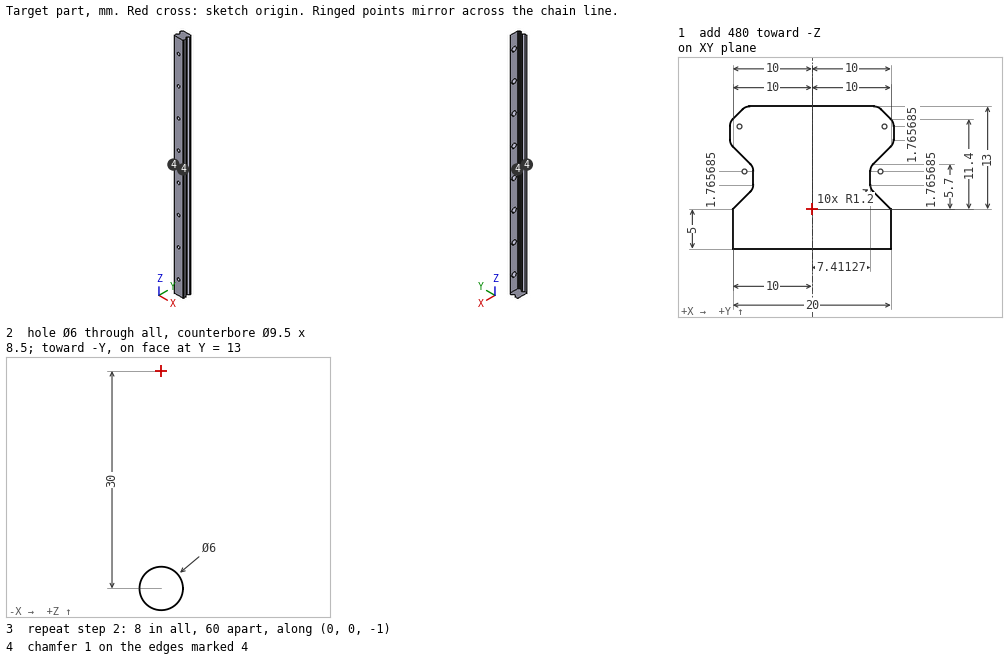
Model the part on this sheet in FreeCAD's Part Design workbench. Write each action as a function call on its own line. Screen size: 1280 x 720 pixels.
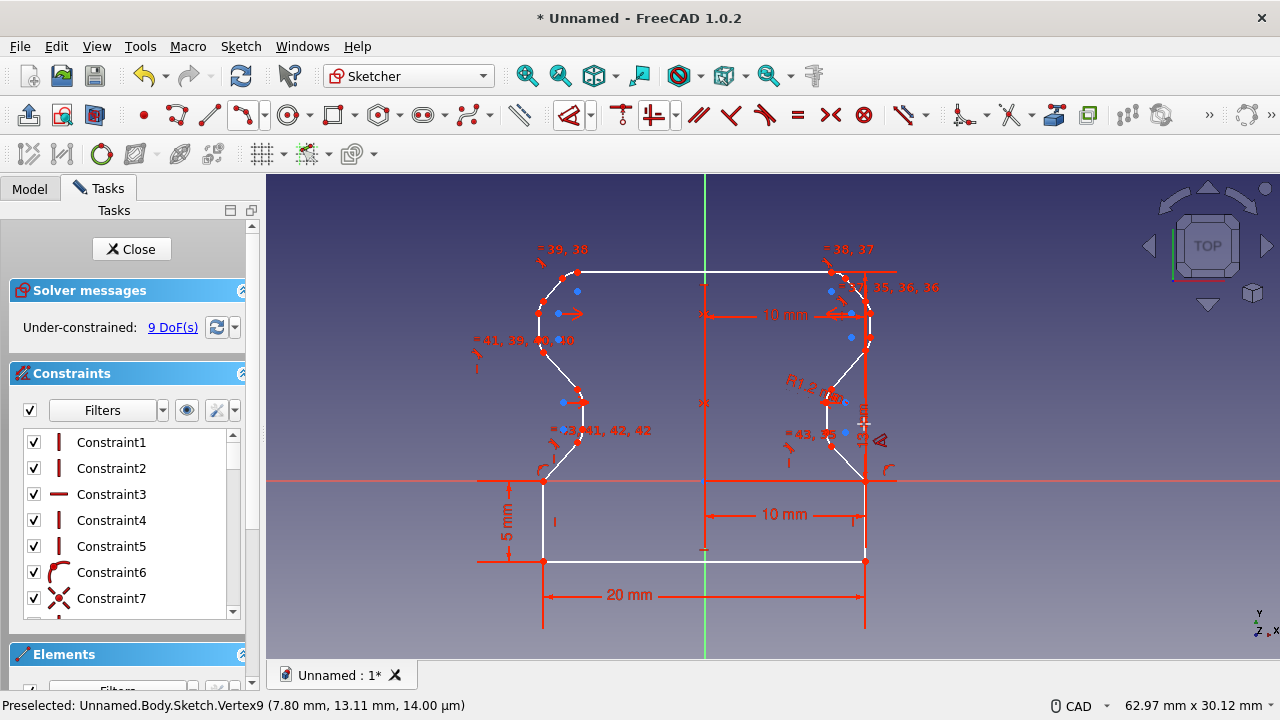
click(543, 301)
click(624, 515)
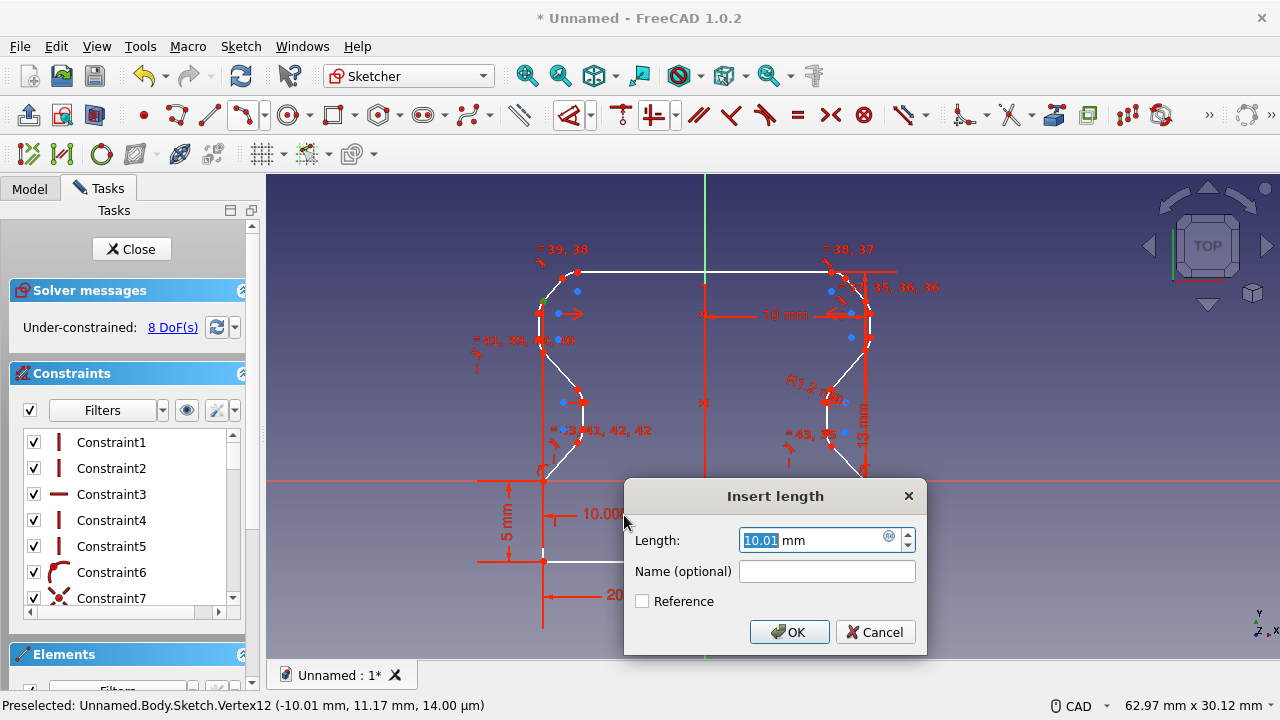
text(10)
key(Return)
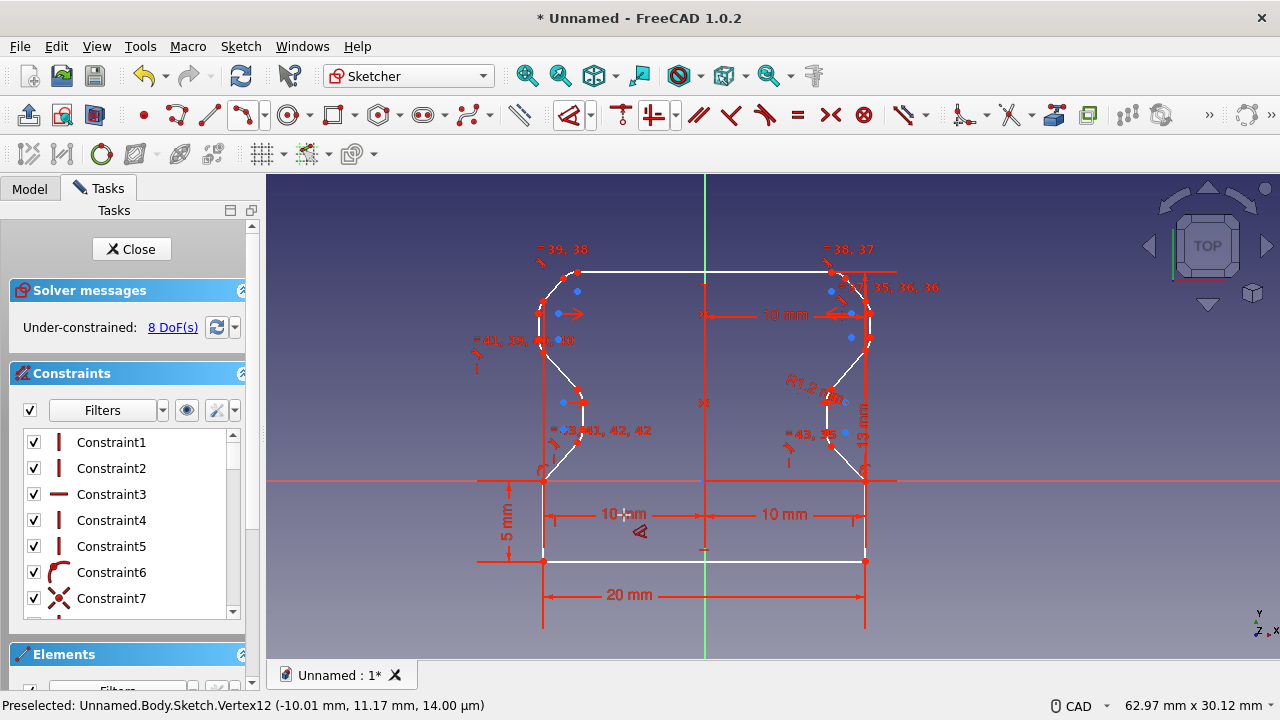
click(544, 352)
click(624, 318)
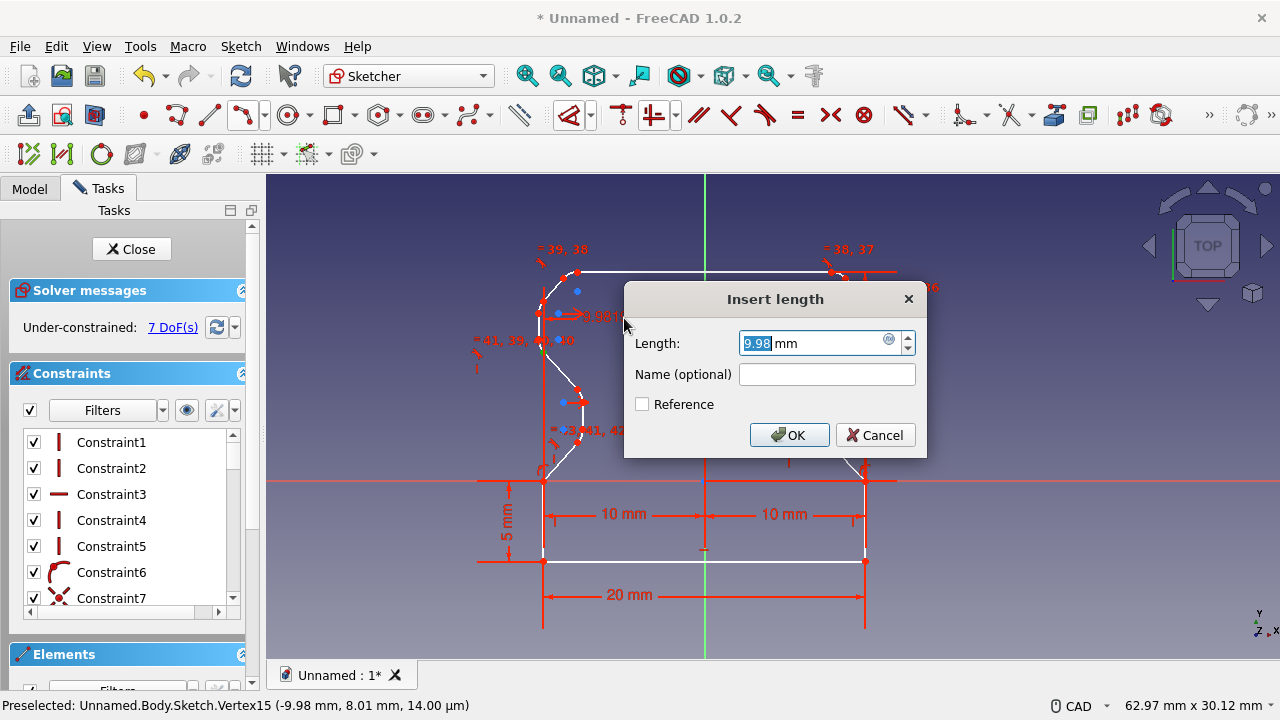
text(10)
key(Return)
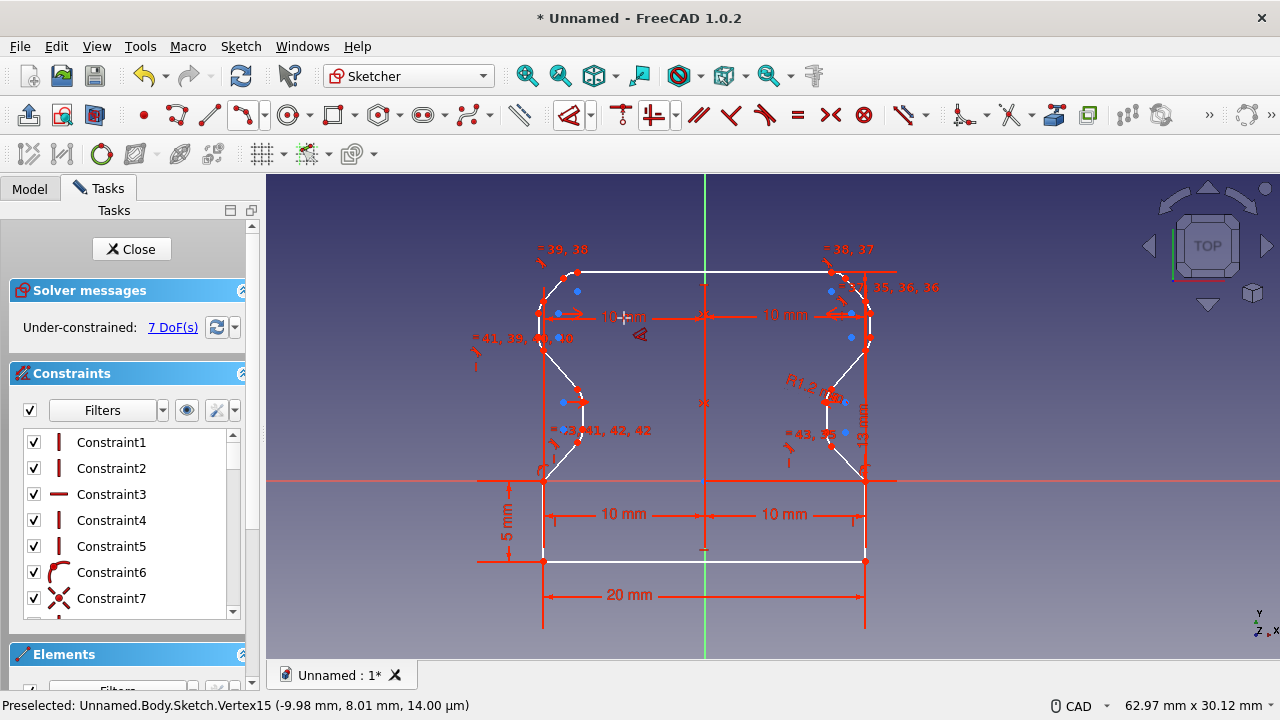
click(543, 481)
click(624, 447)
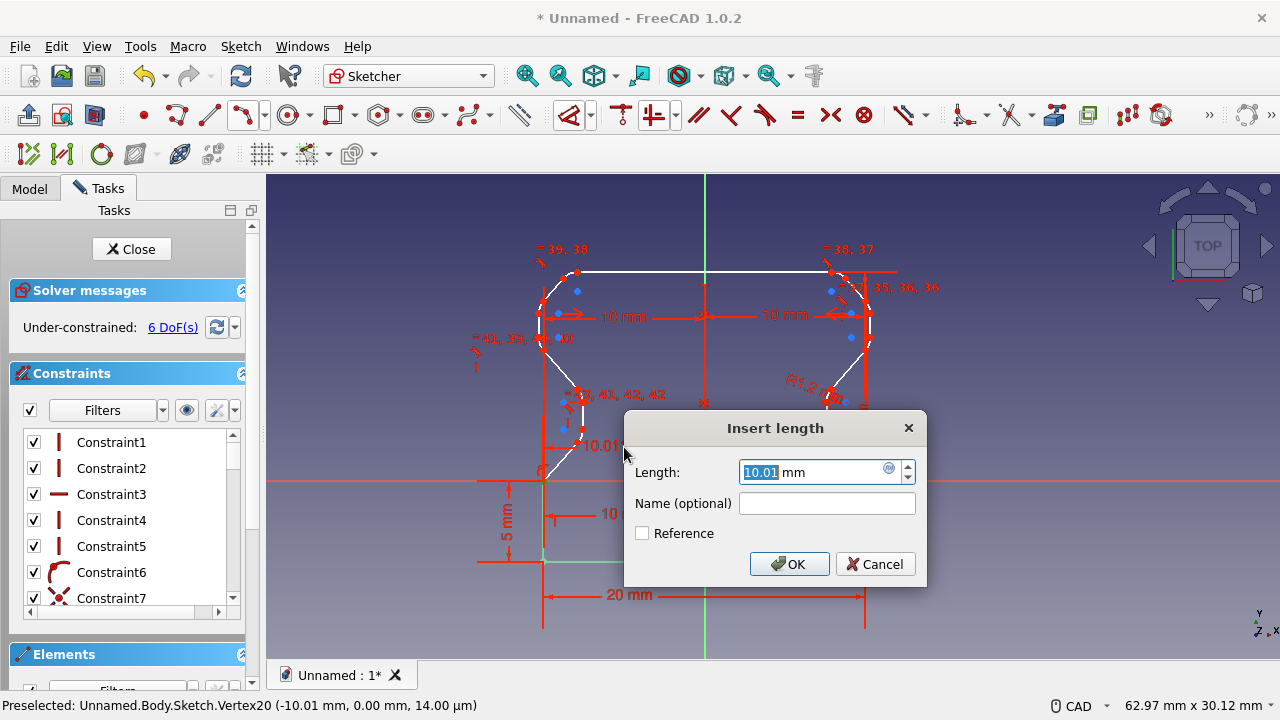
text(10)
key(Return)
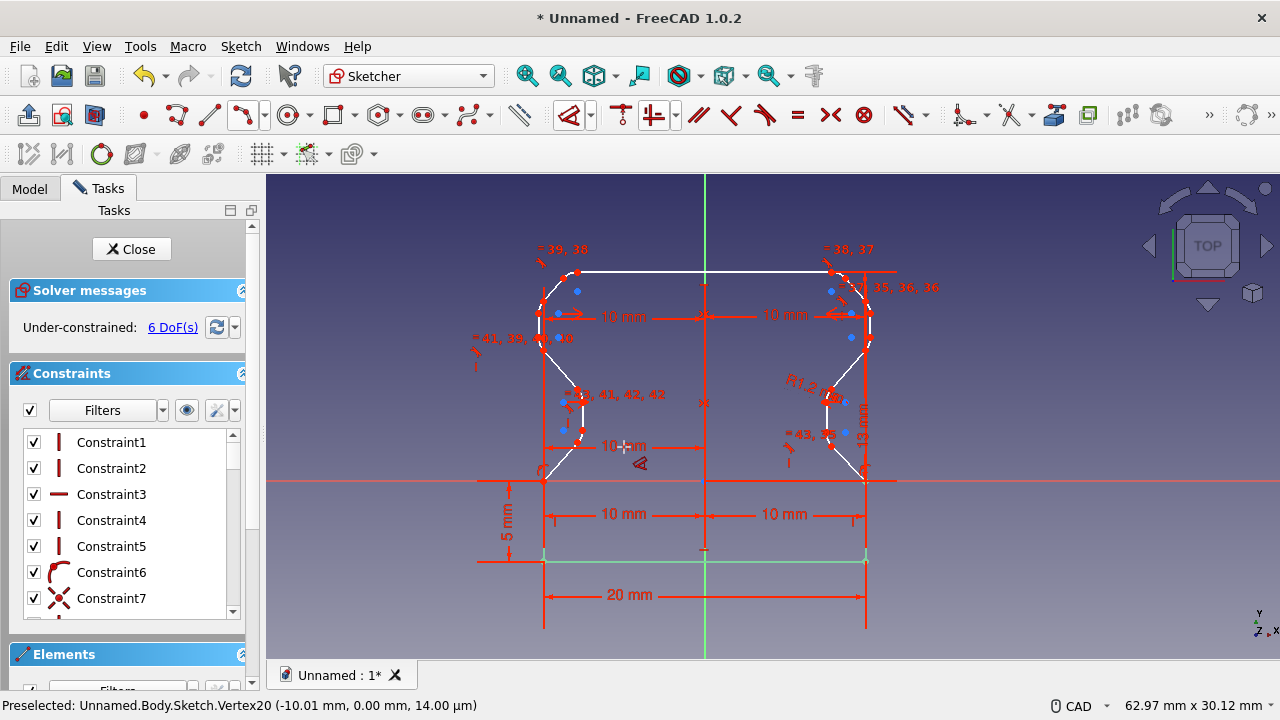
click(831, 390)
click(865, 457)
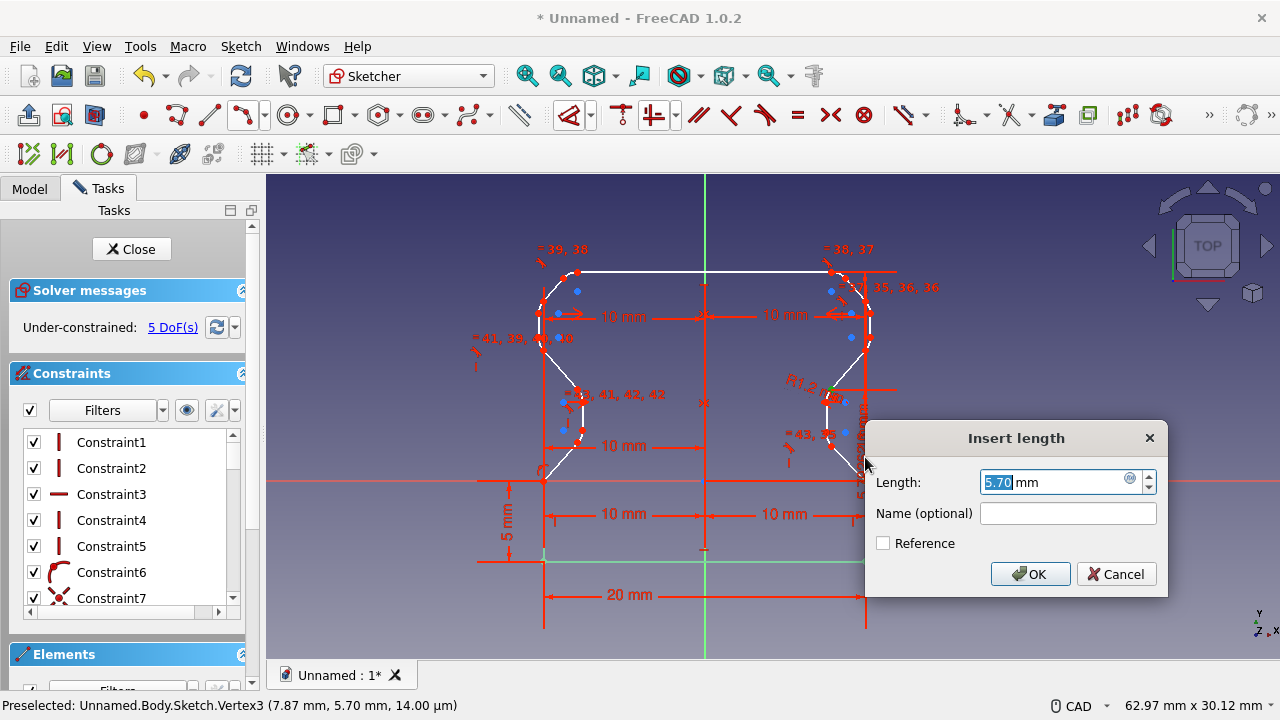
text(5.7)
key(Return)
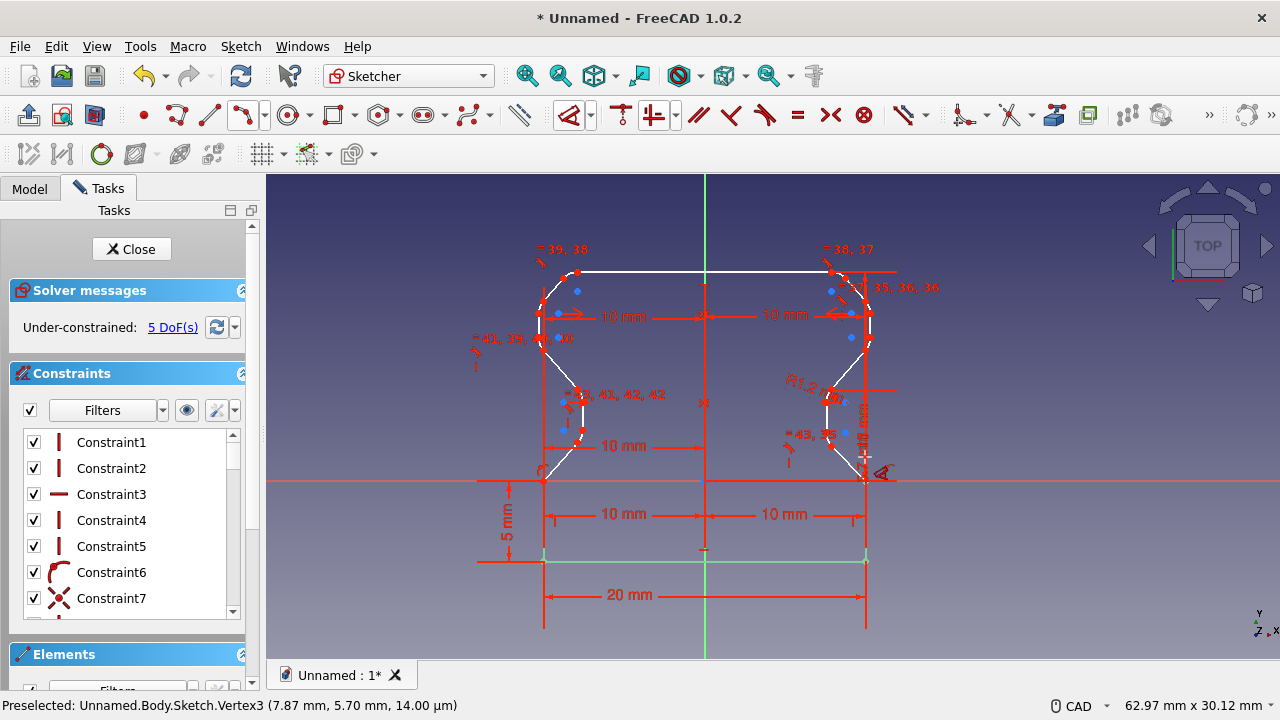
click(866, 301)
click(900, 391)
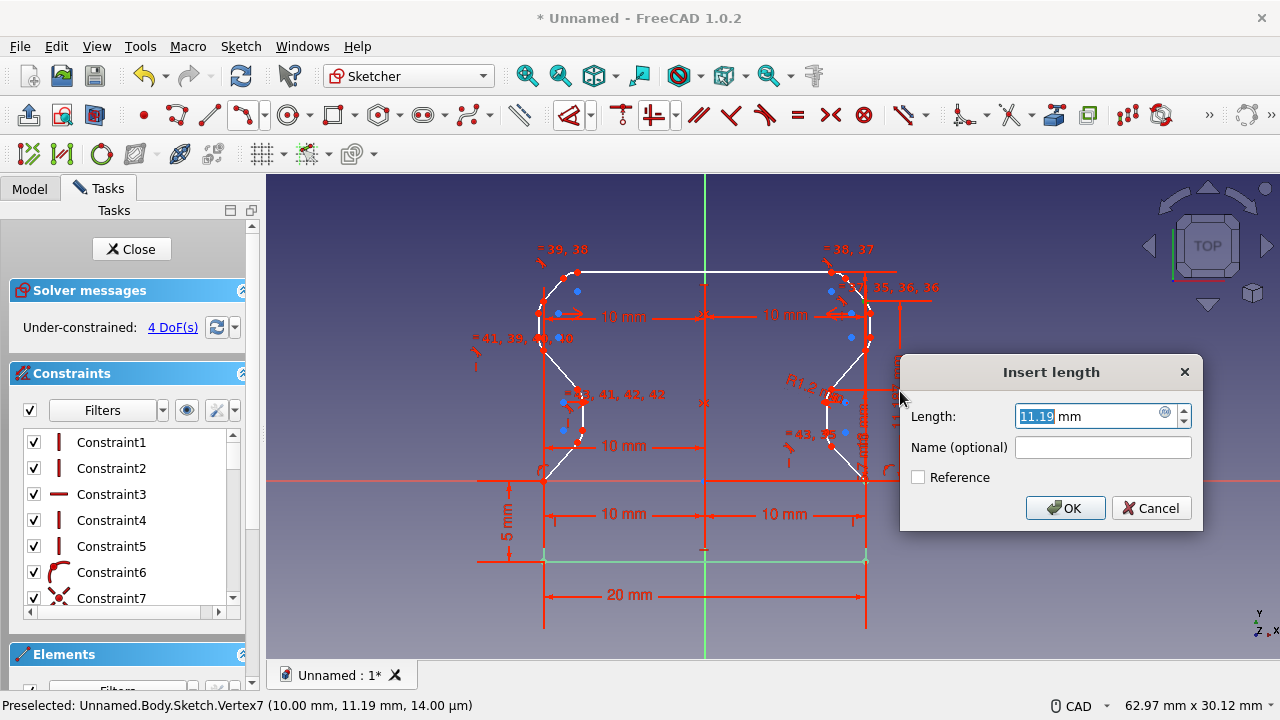
text(11.4)
key(Return)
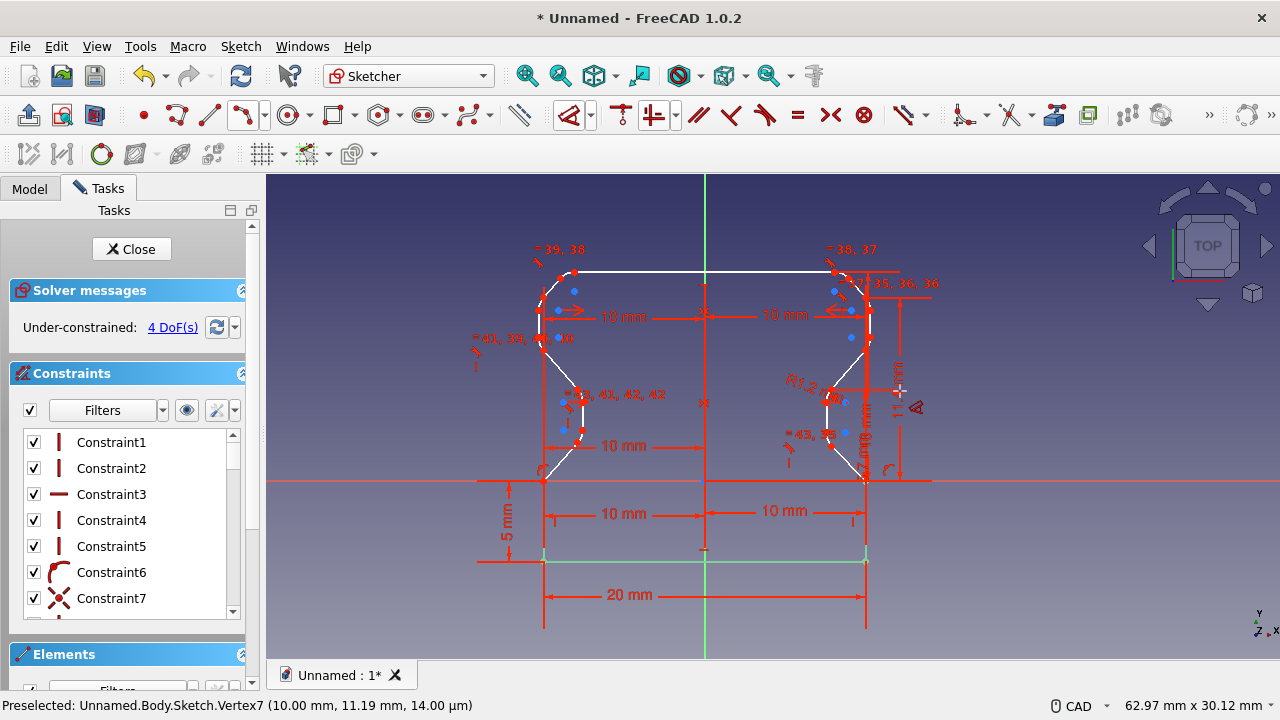
scroll(827, 424, up, 3)